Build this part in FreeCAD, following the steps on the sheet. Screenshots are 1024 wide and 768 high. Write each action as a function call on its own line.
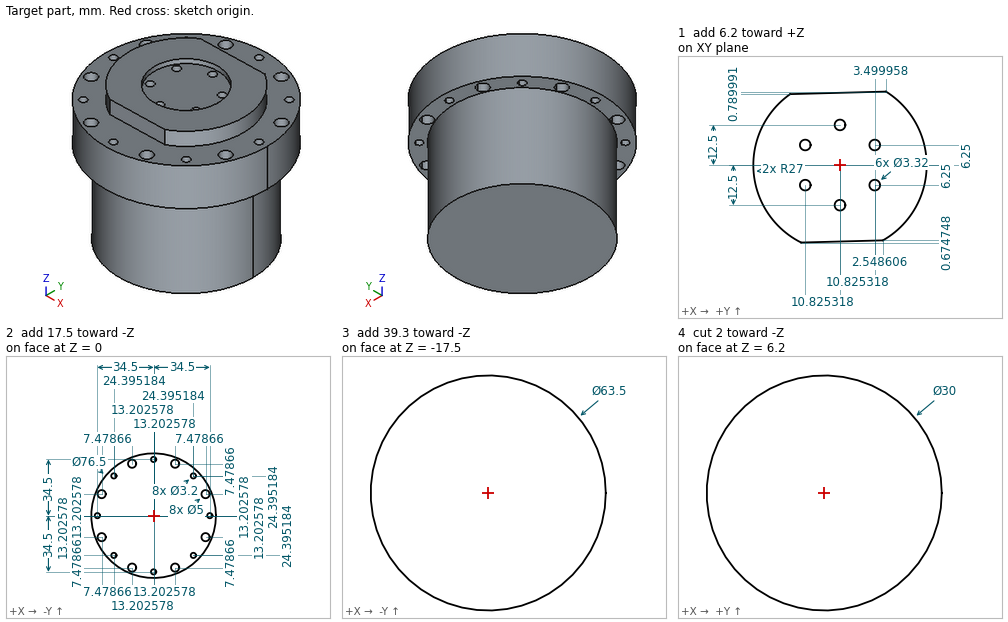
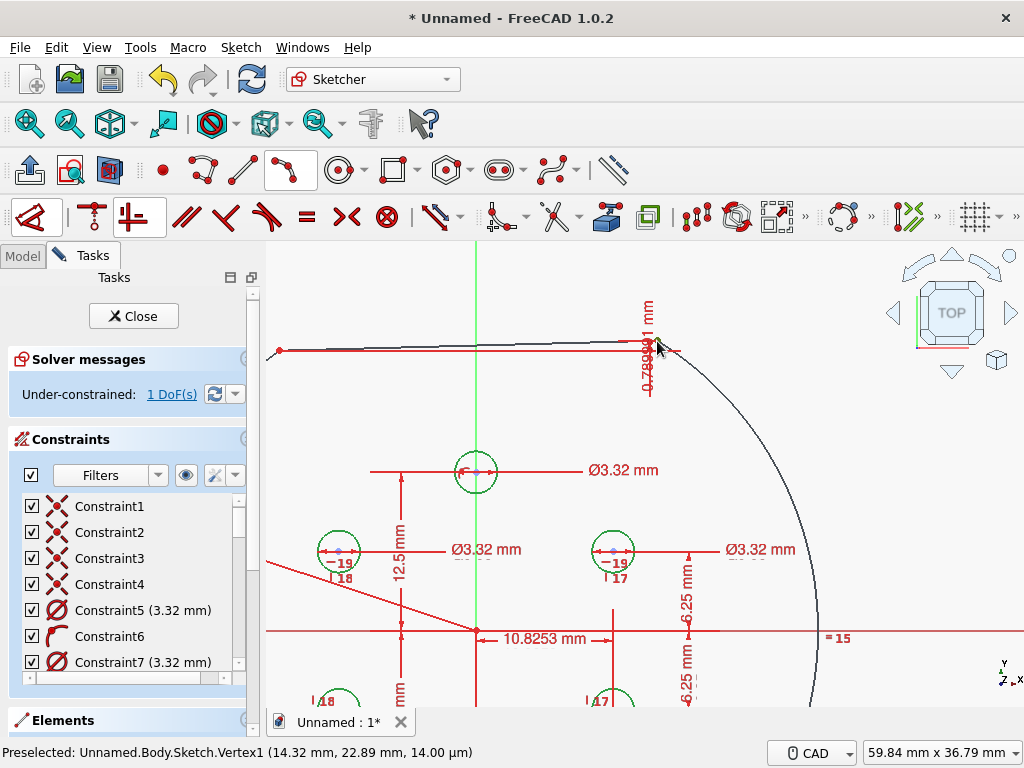
scroll(658, 340, down, 4)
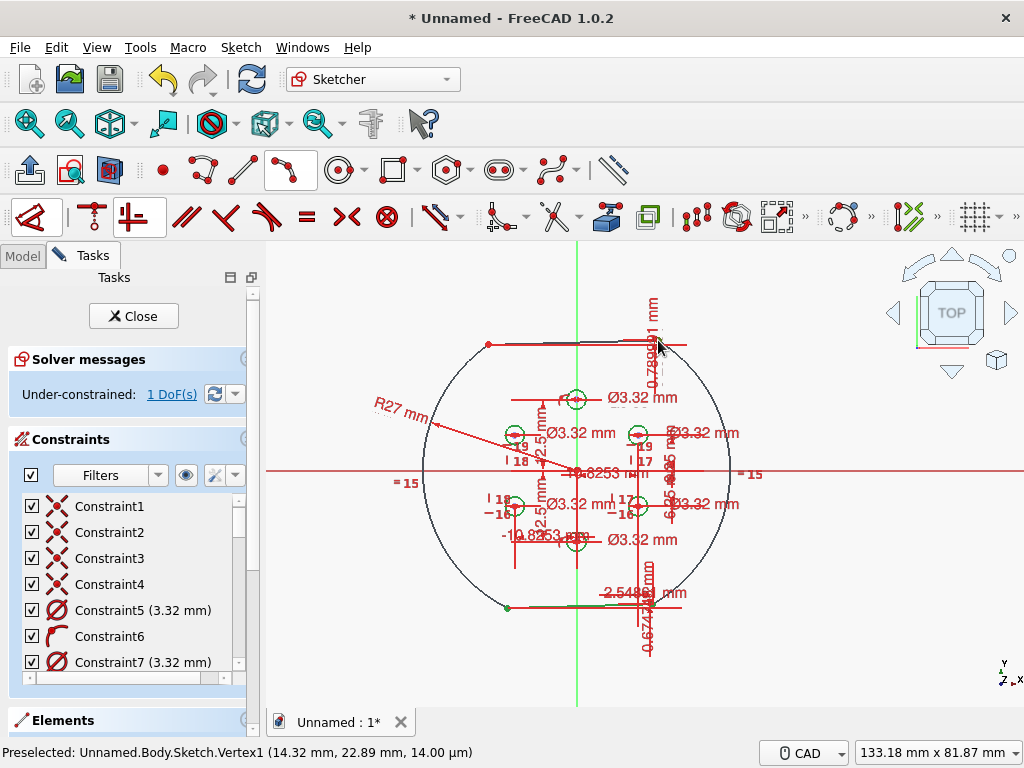
scroll(638, 506, up, 4)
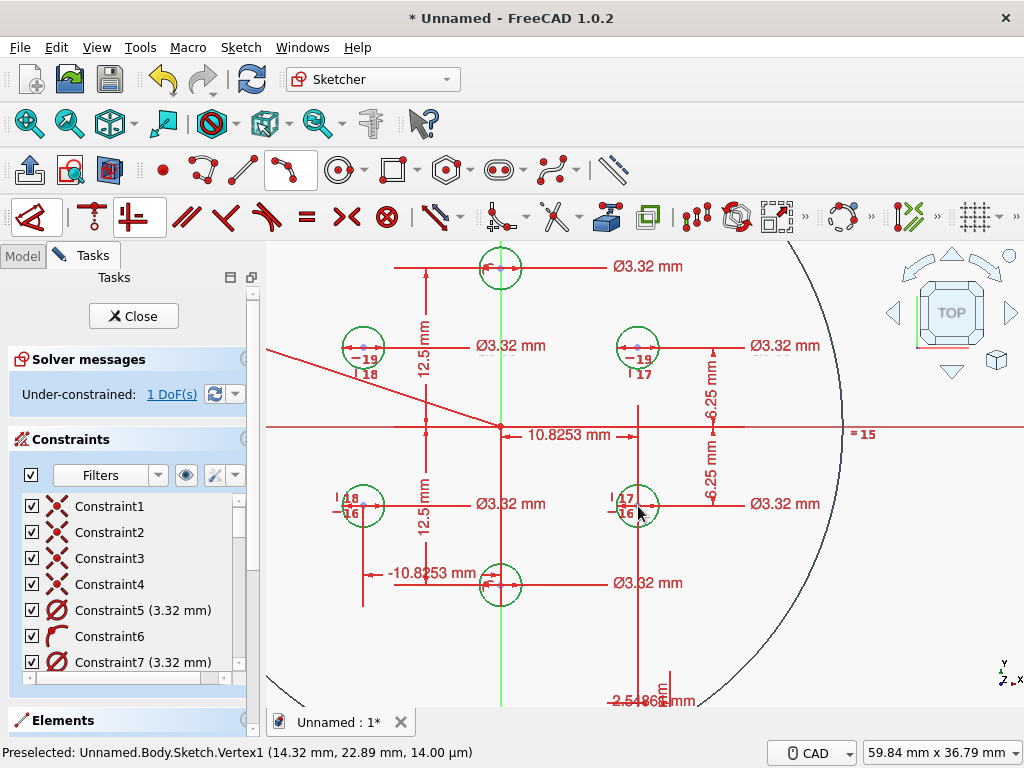
click(638, 506)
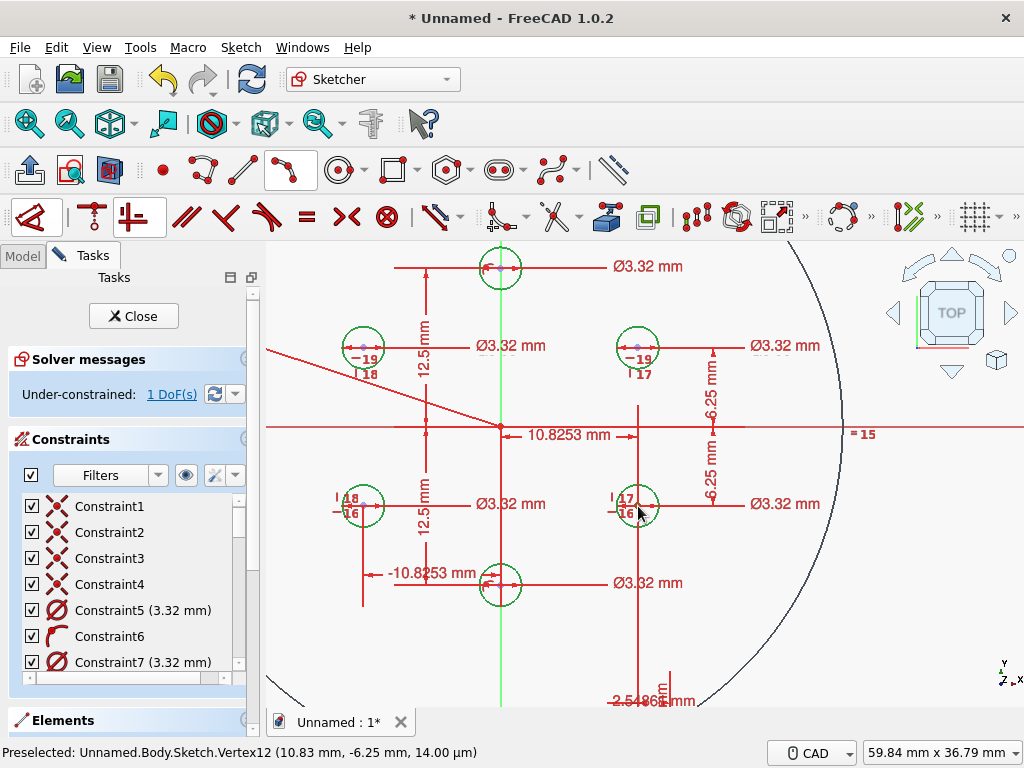
key(l)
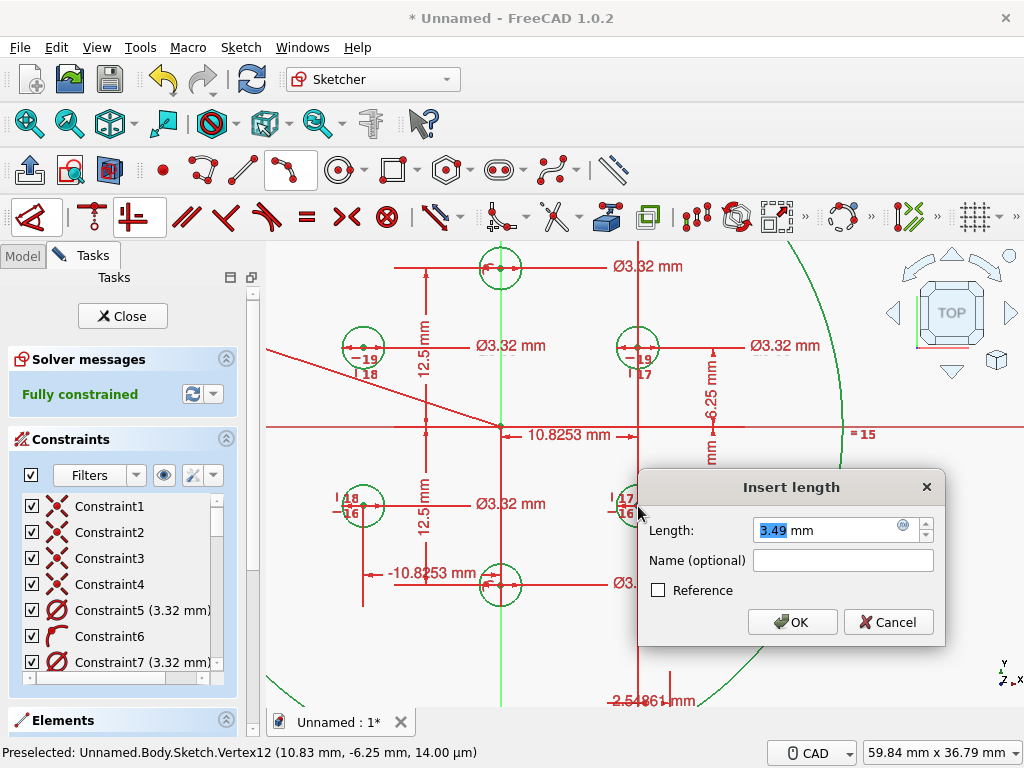
text(3.499958)
key(Return)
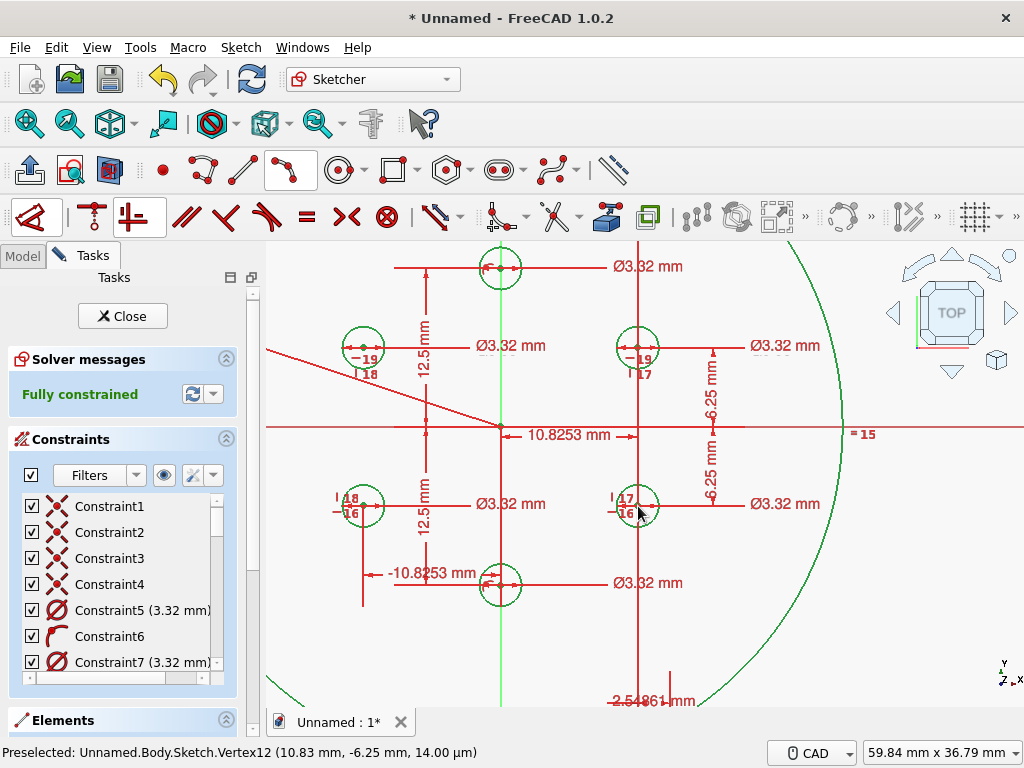
click(123, 316)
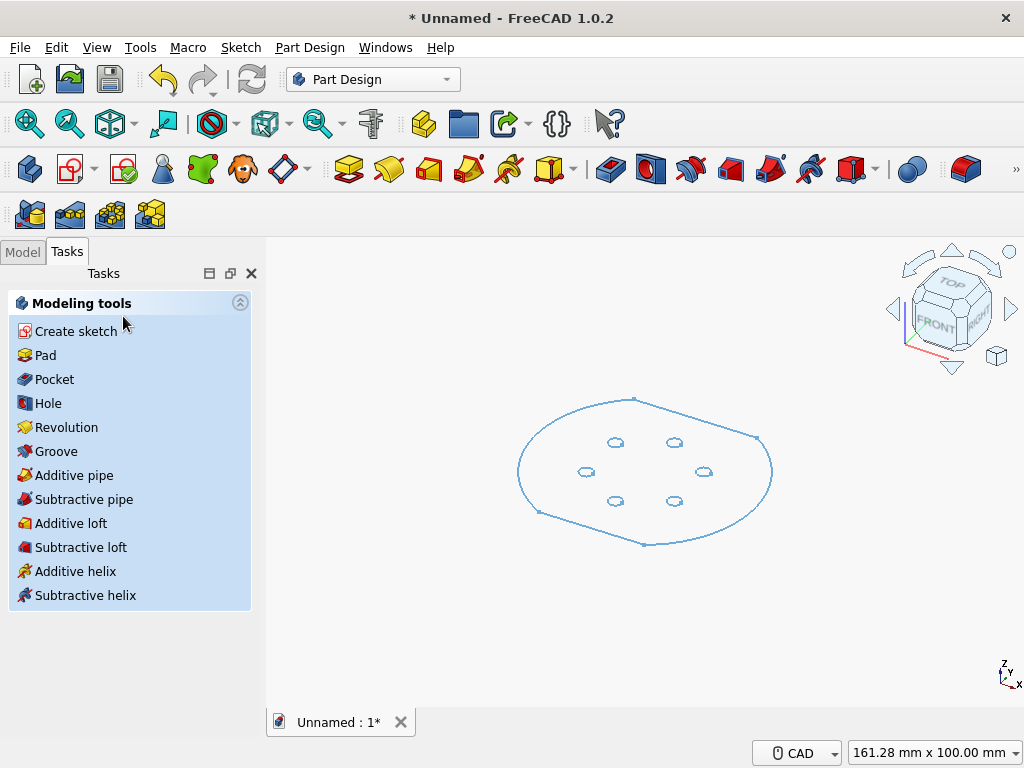
click(350, 170)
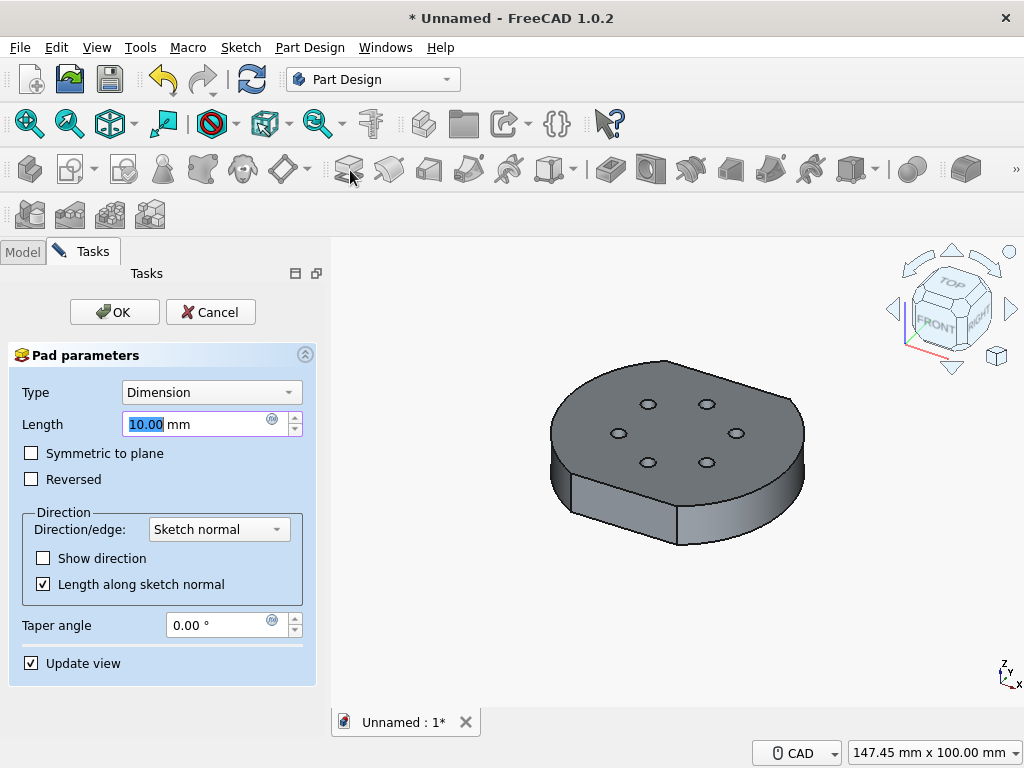
text(6.2)
key(Tab)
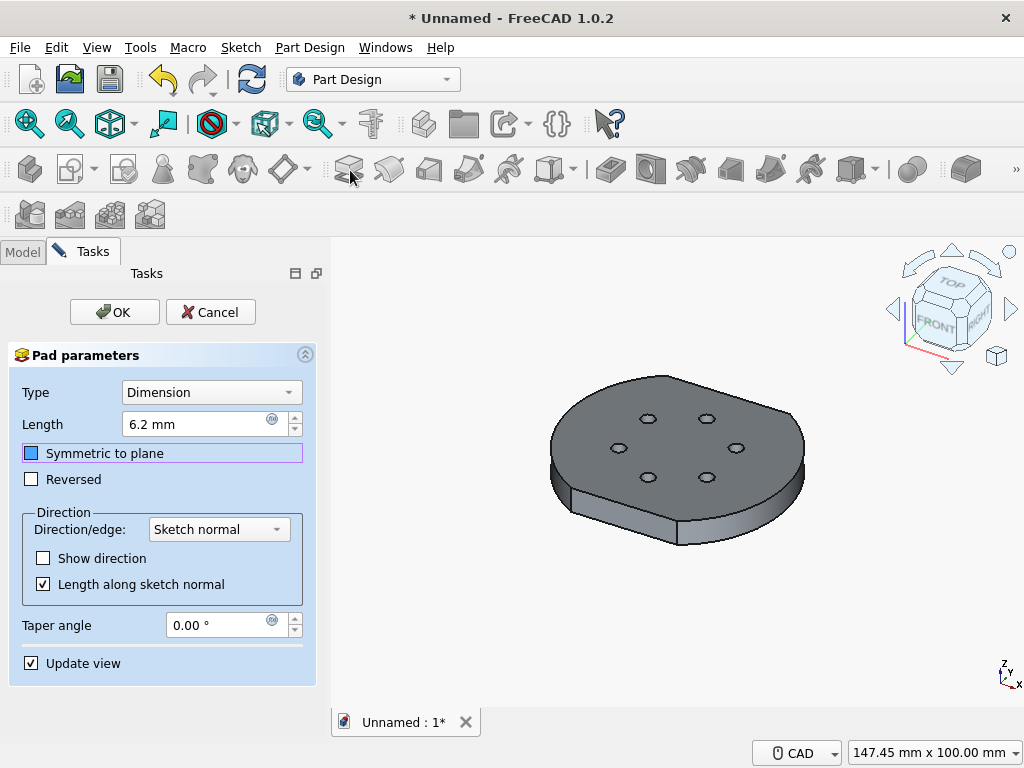
click(115, 312)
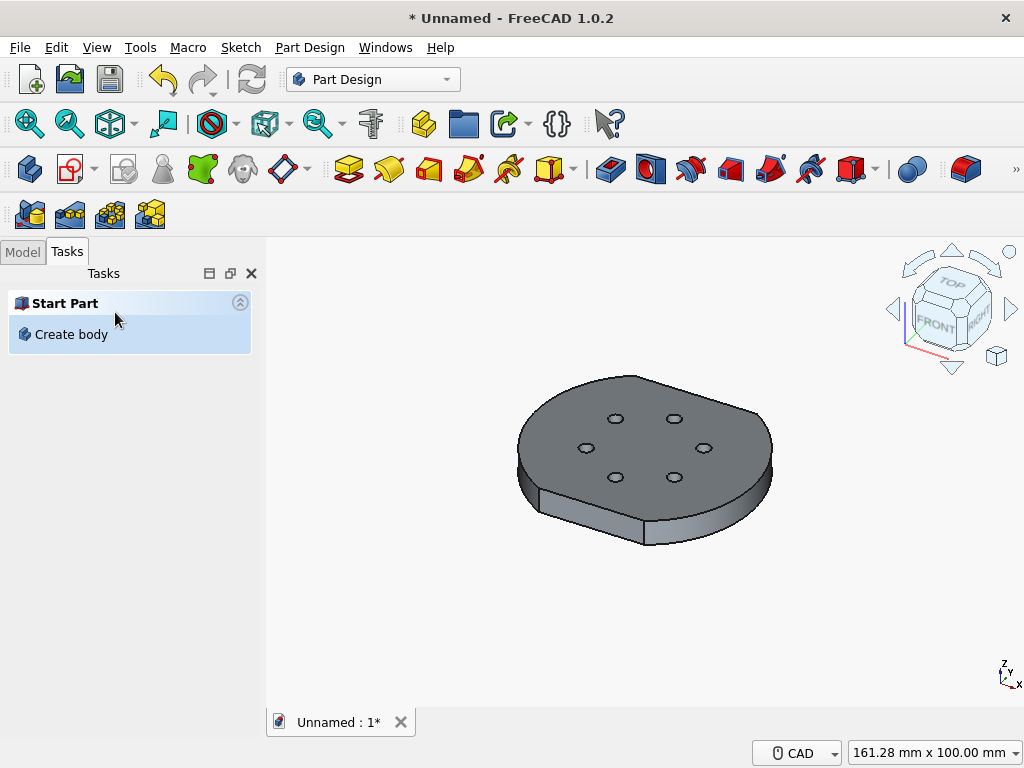
click(30, 124)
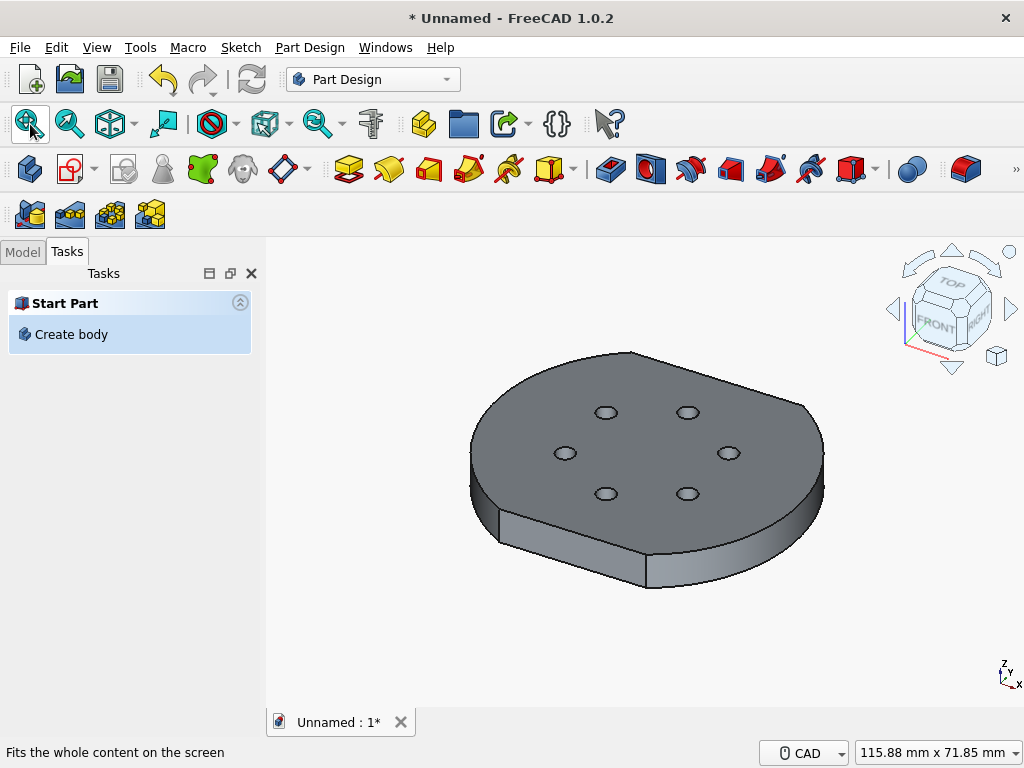
key(5)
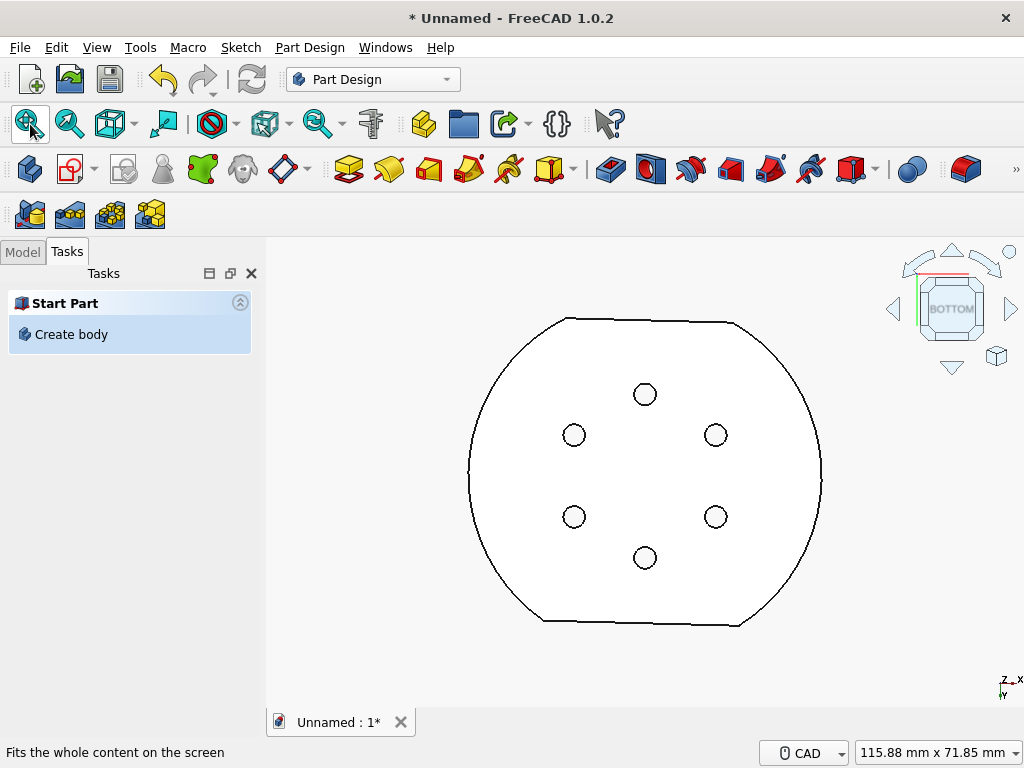
click(645, 471)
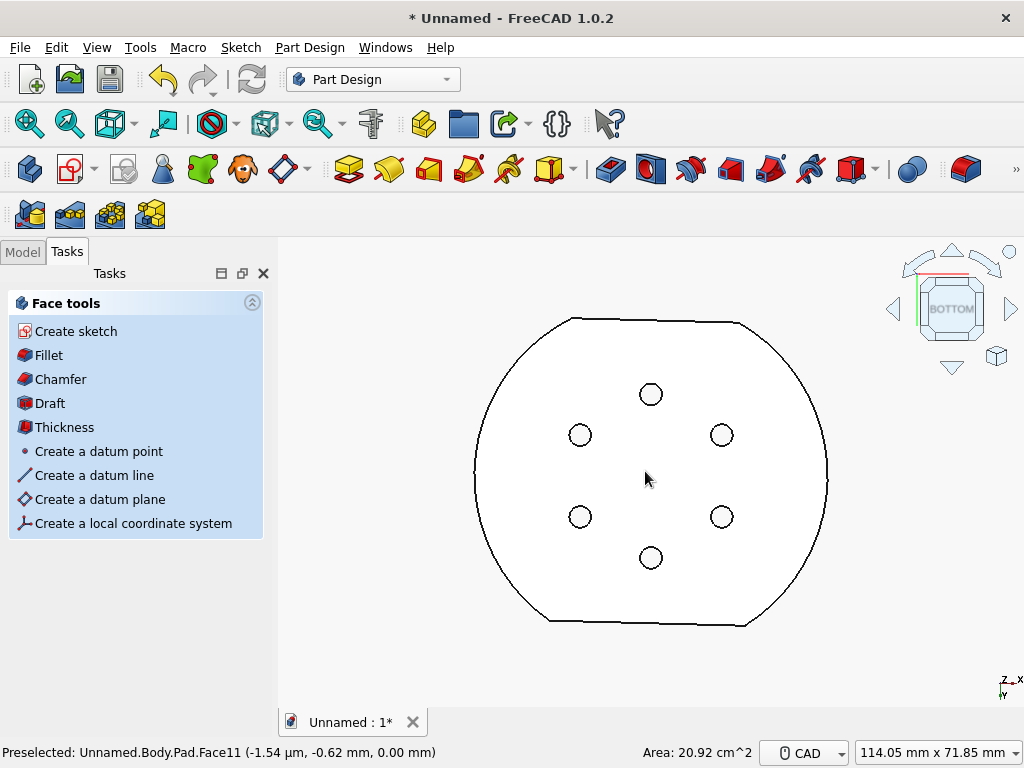
click(70, 170)